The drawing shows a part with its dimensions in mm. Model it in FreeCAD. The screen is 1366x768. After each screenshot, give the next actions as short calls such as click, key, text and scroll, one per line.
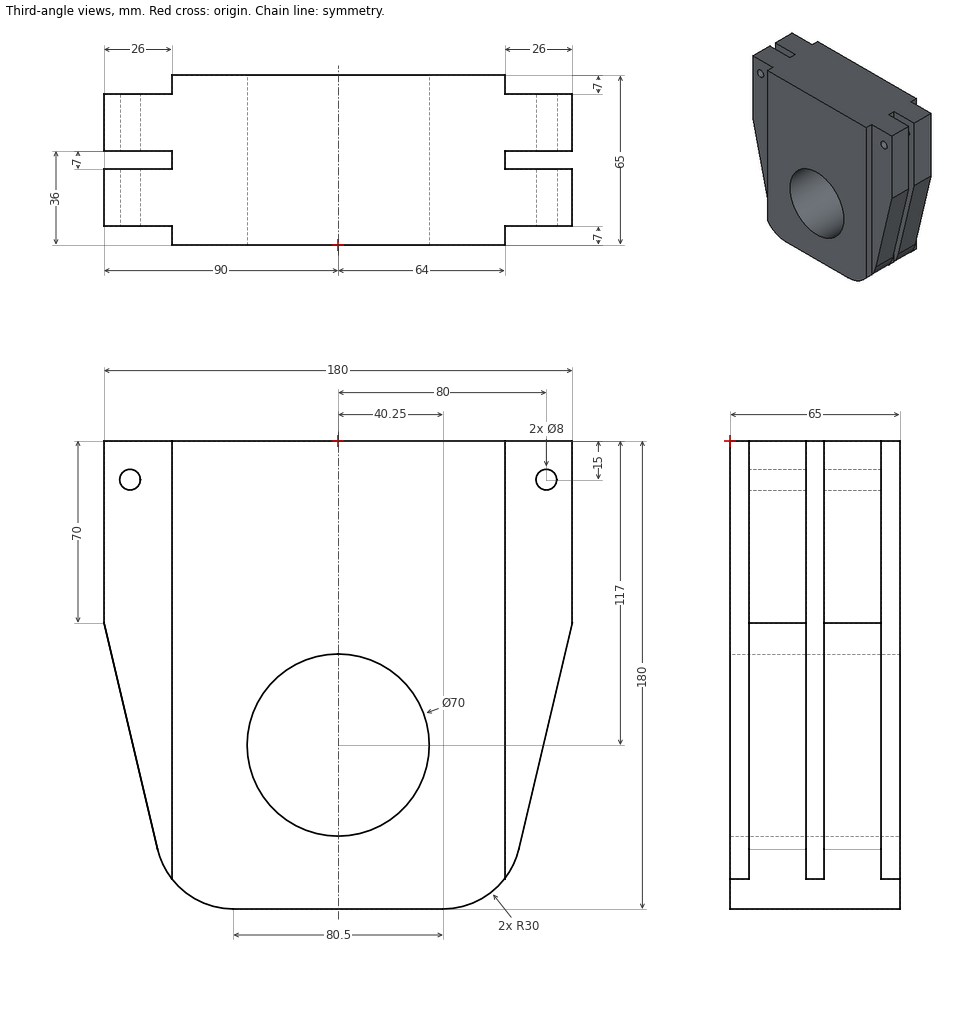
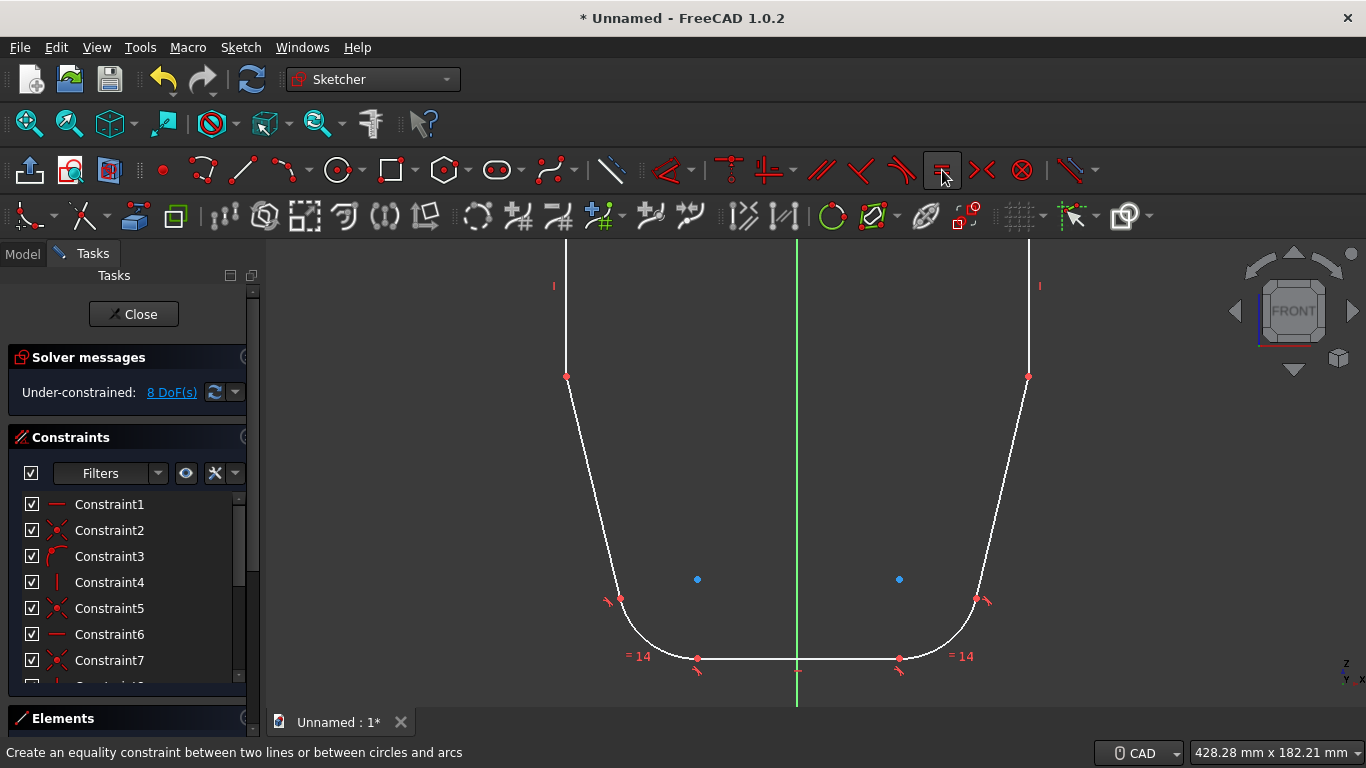
click(566, 376)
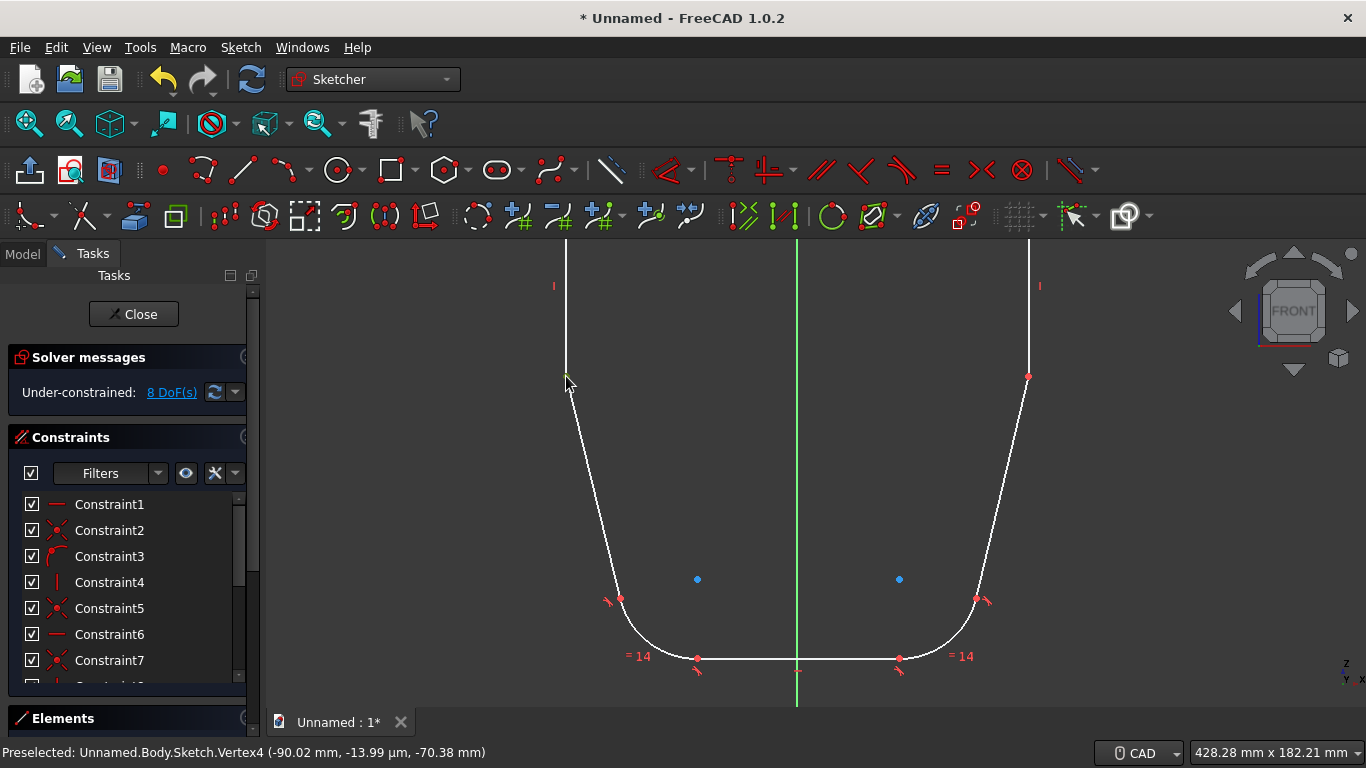
click(1029, 376)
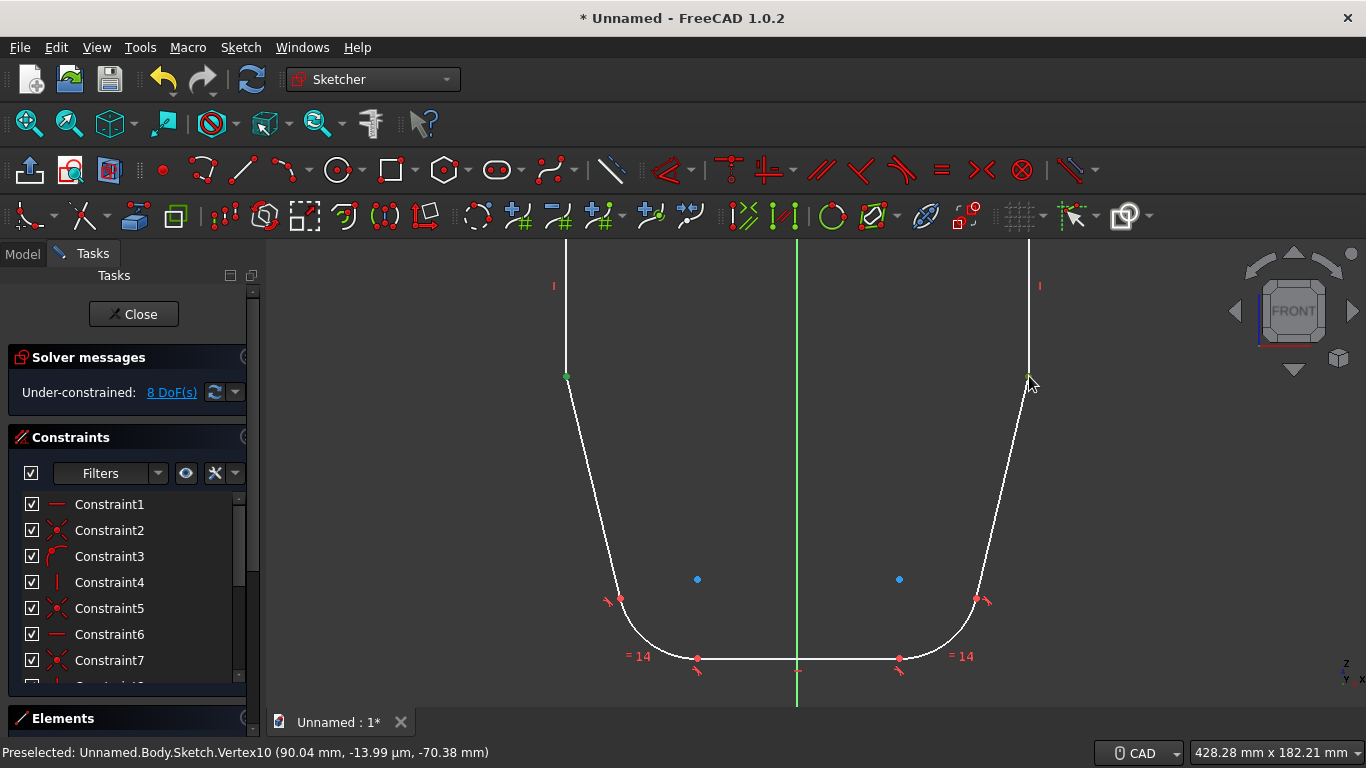
click(797, 620)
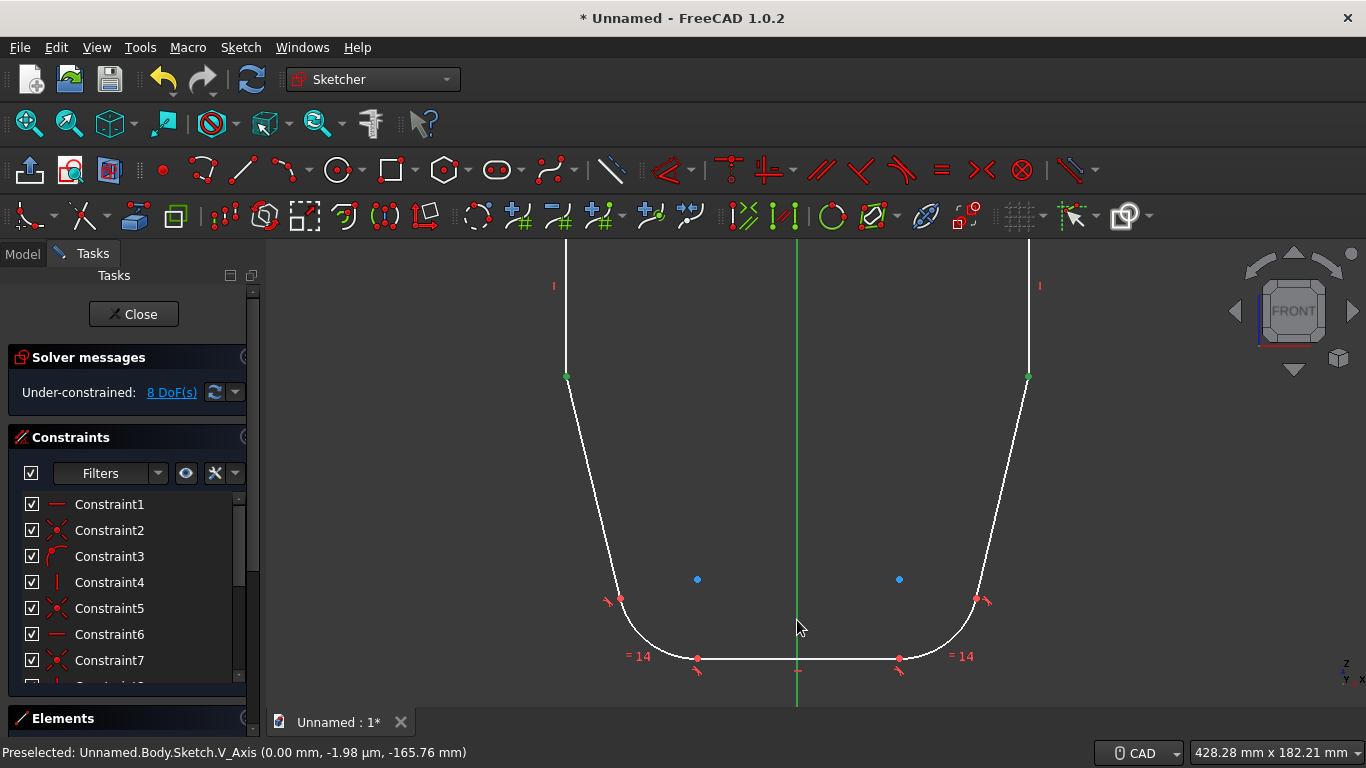
click(982, 170)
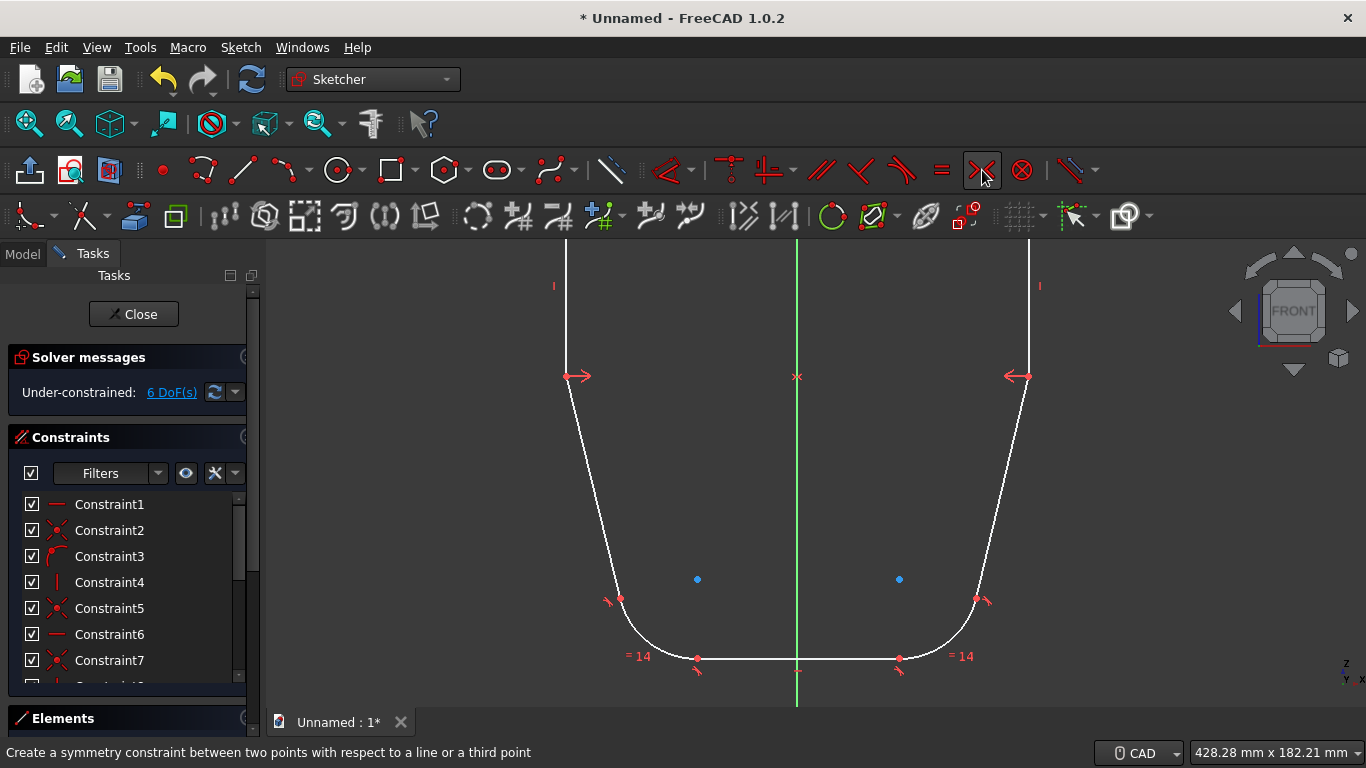
click(634, 627)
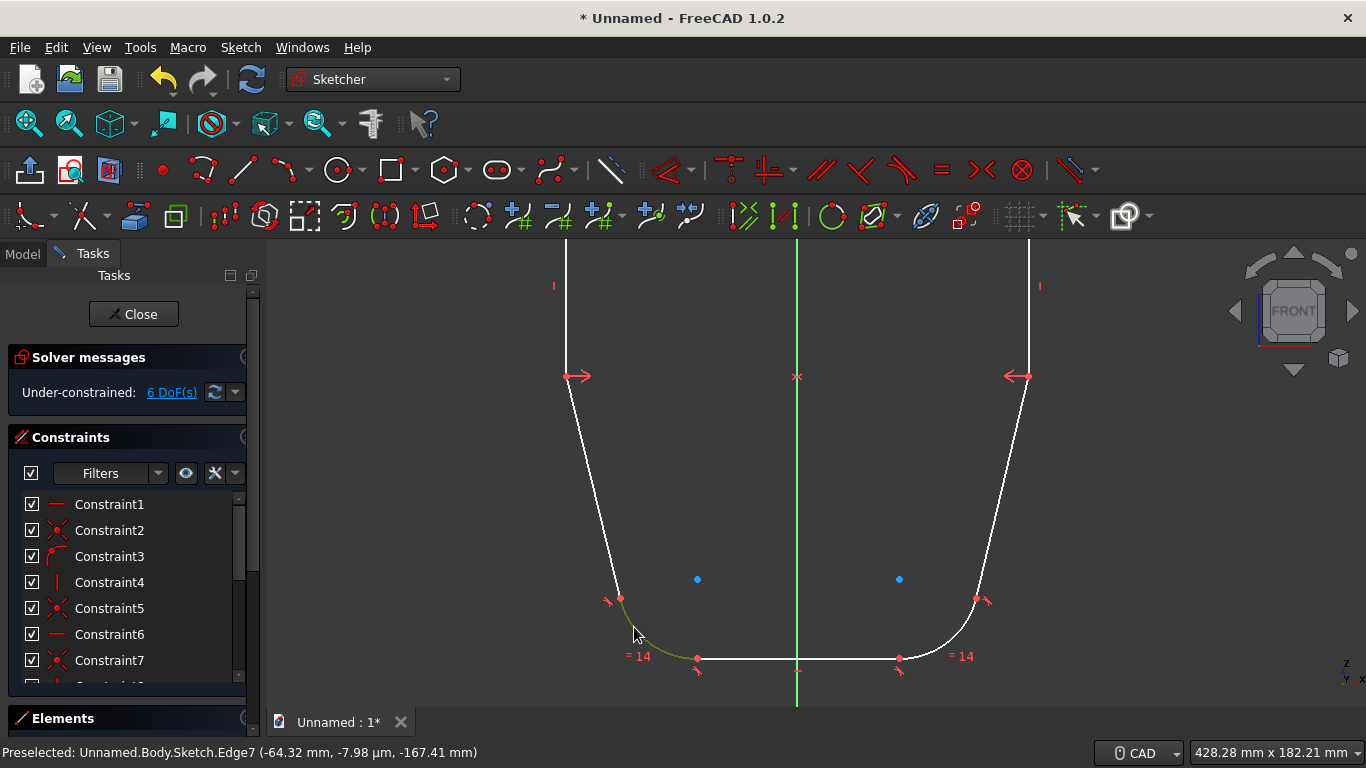
click(694, 170)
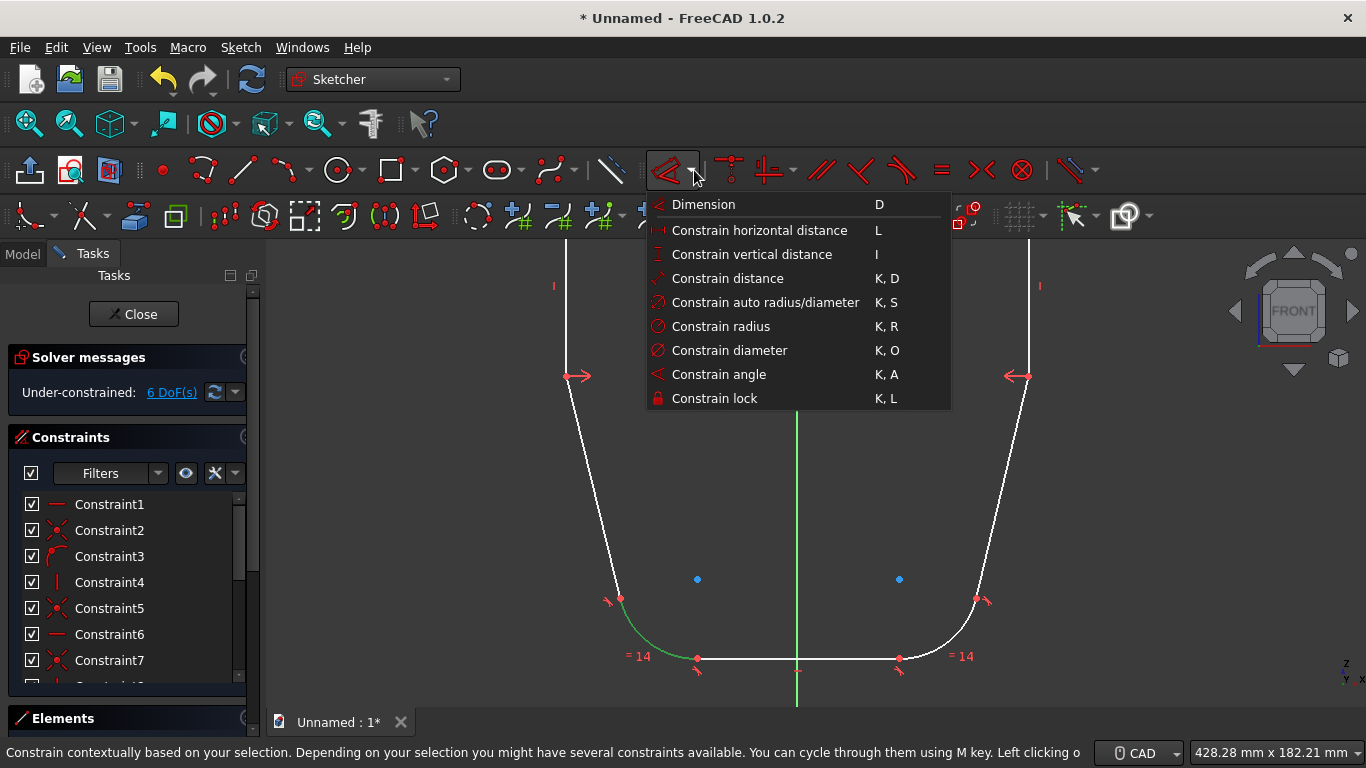
click(799, 326)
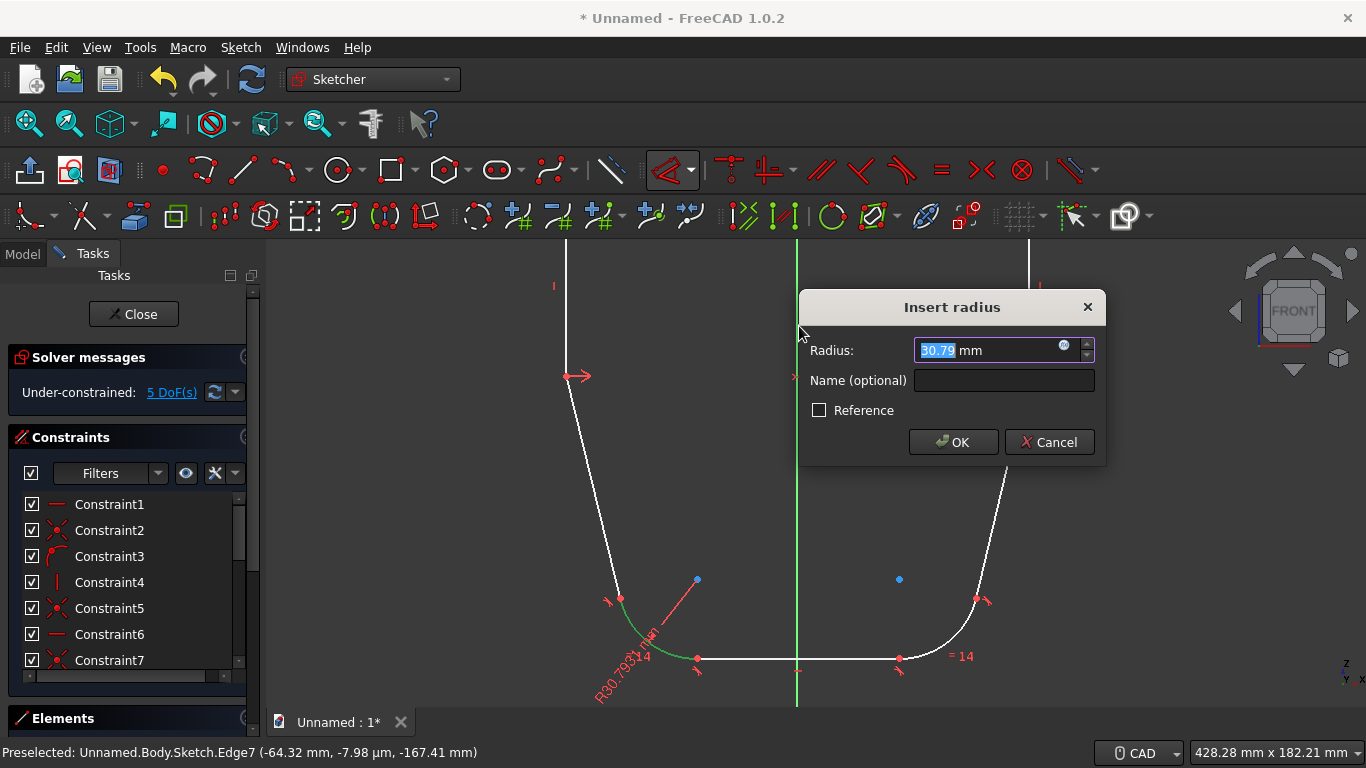
text(30)
key(Return)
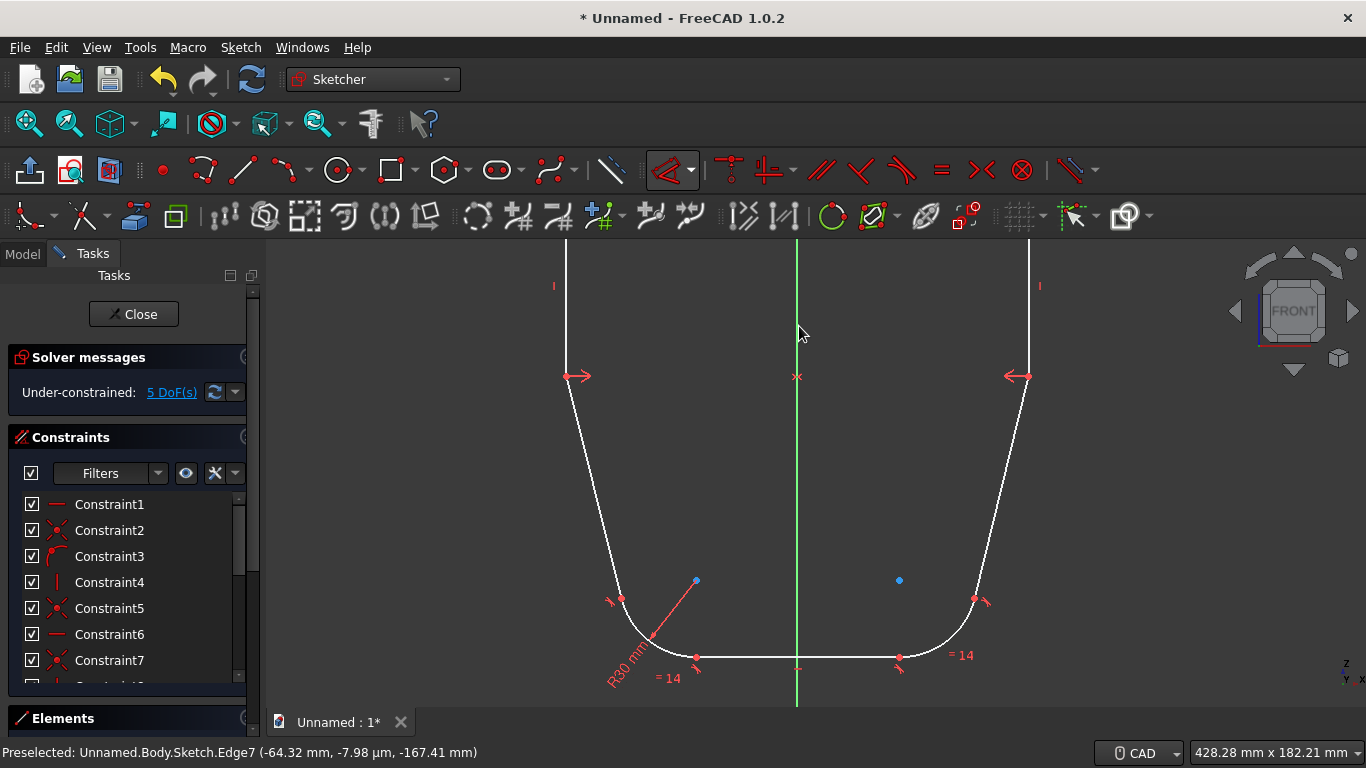
click(566, 322)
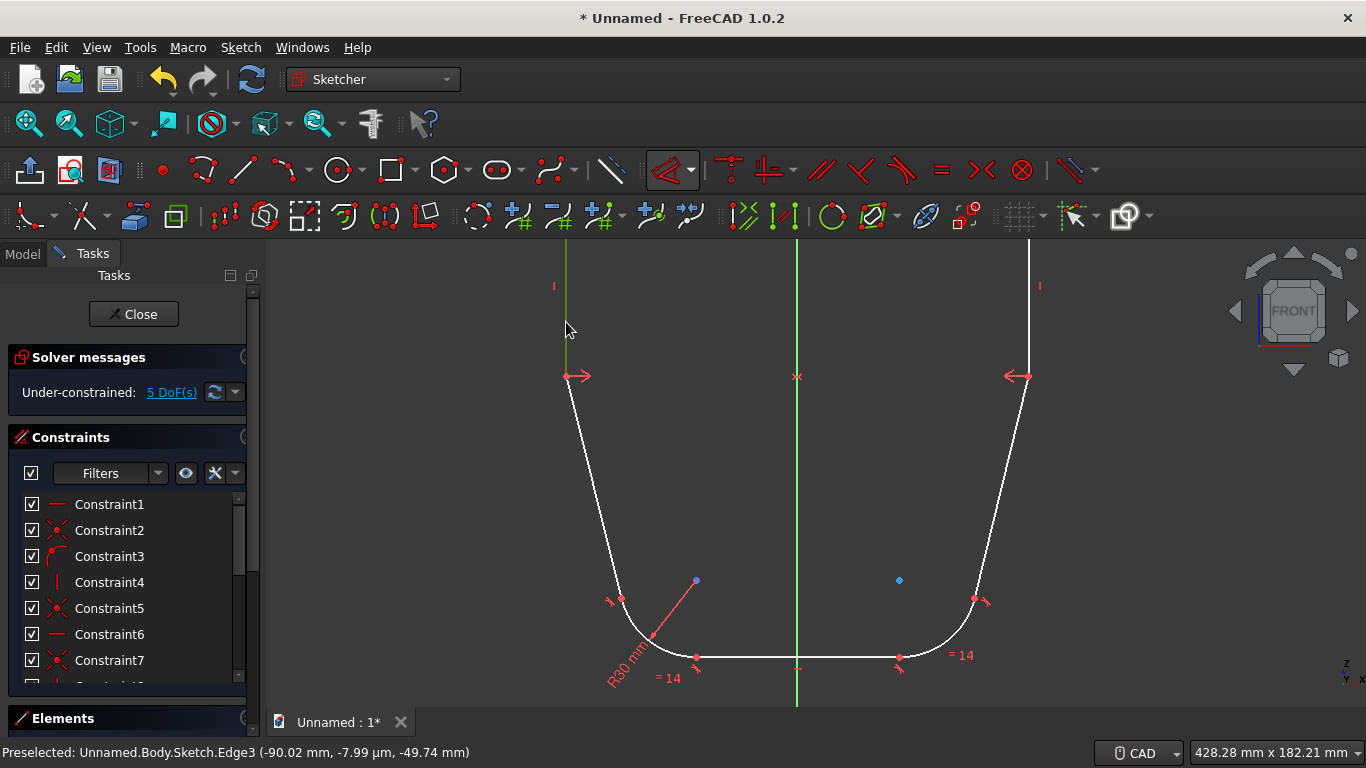
click(694, 170)